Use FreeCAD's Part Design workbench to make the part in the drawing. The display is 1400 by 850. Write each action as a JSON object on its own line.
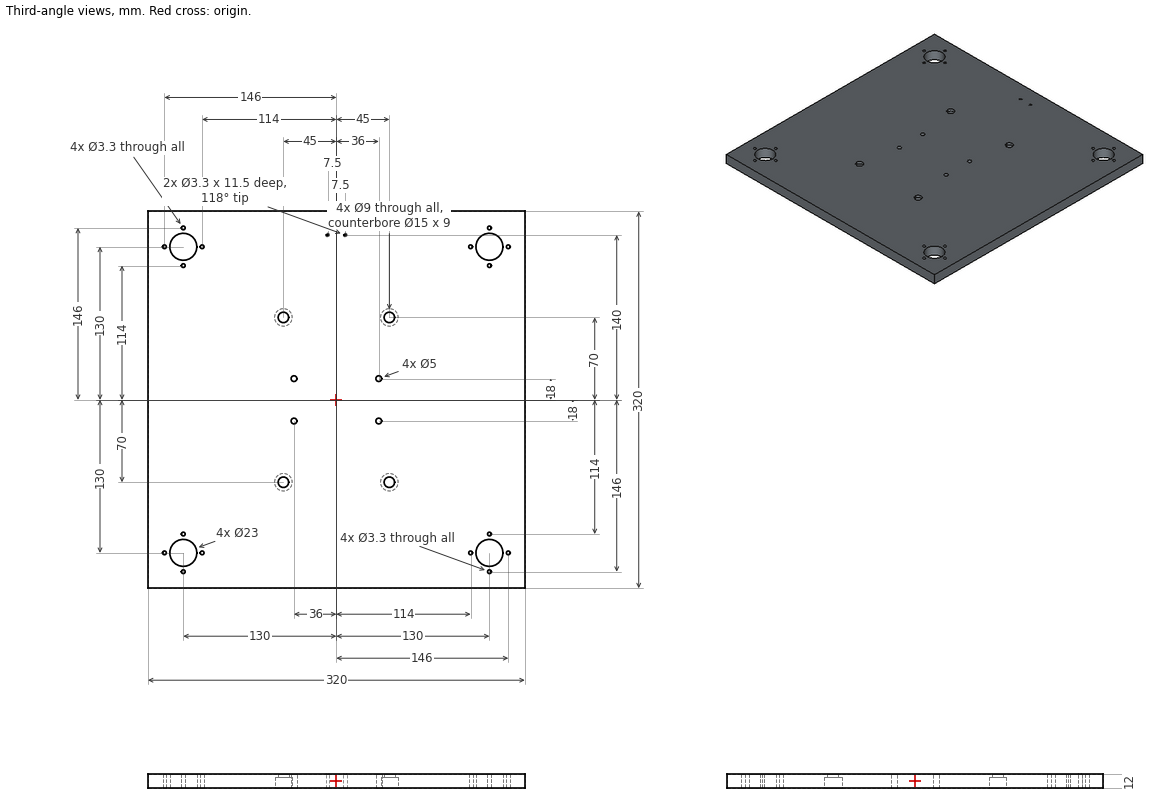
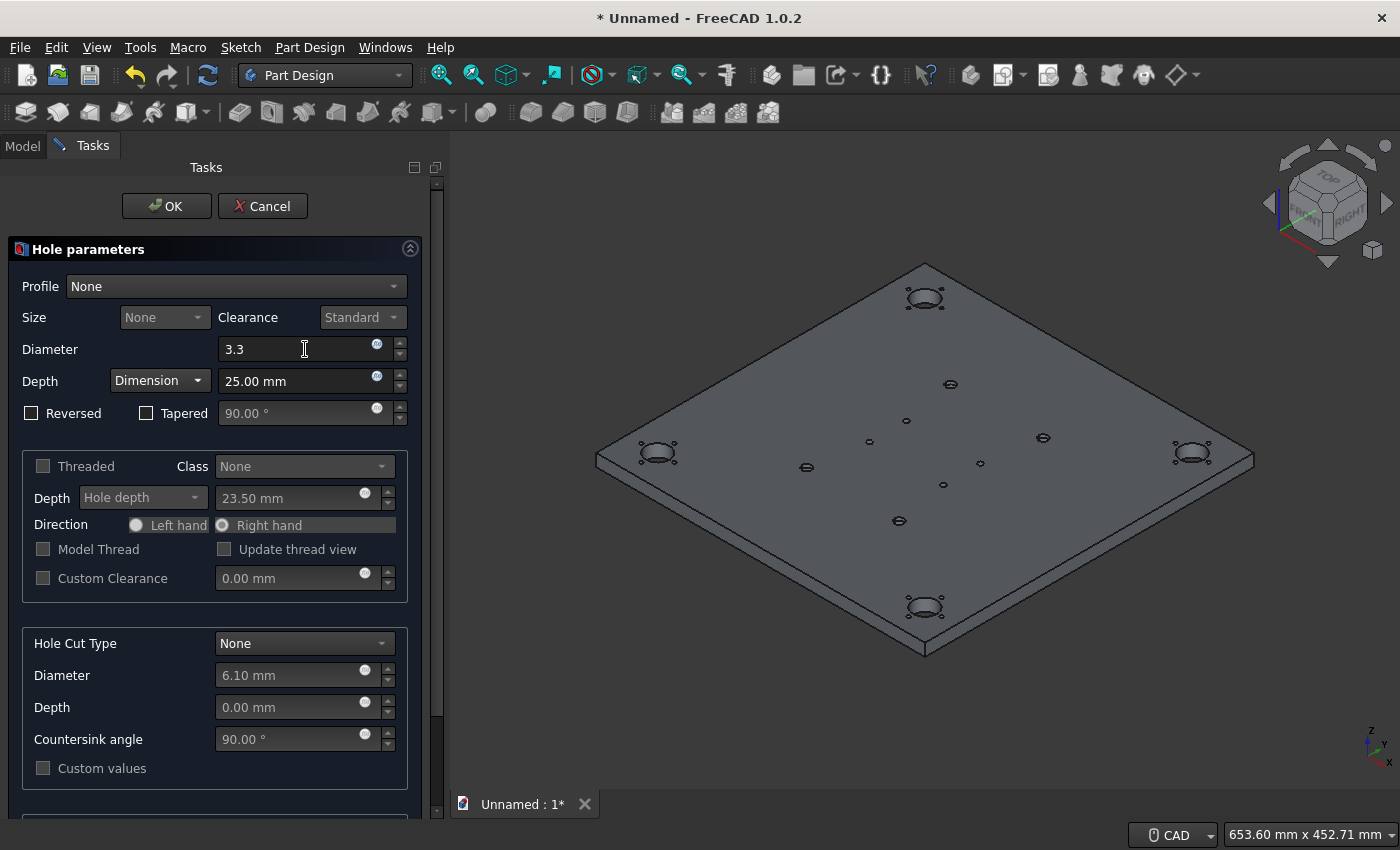
{"action": "left_click", "coordinate": [161, 380]}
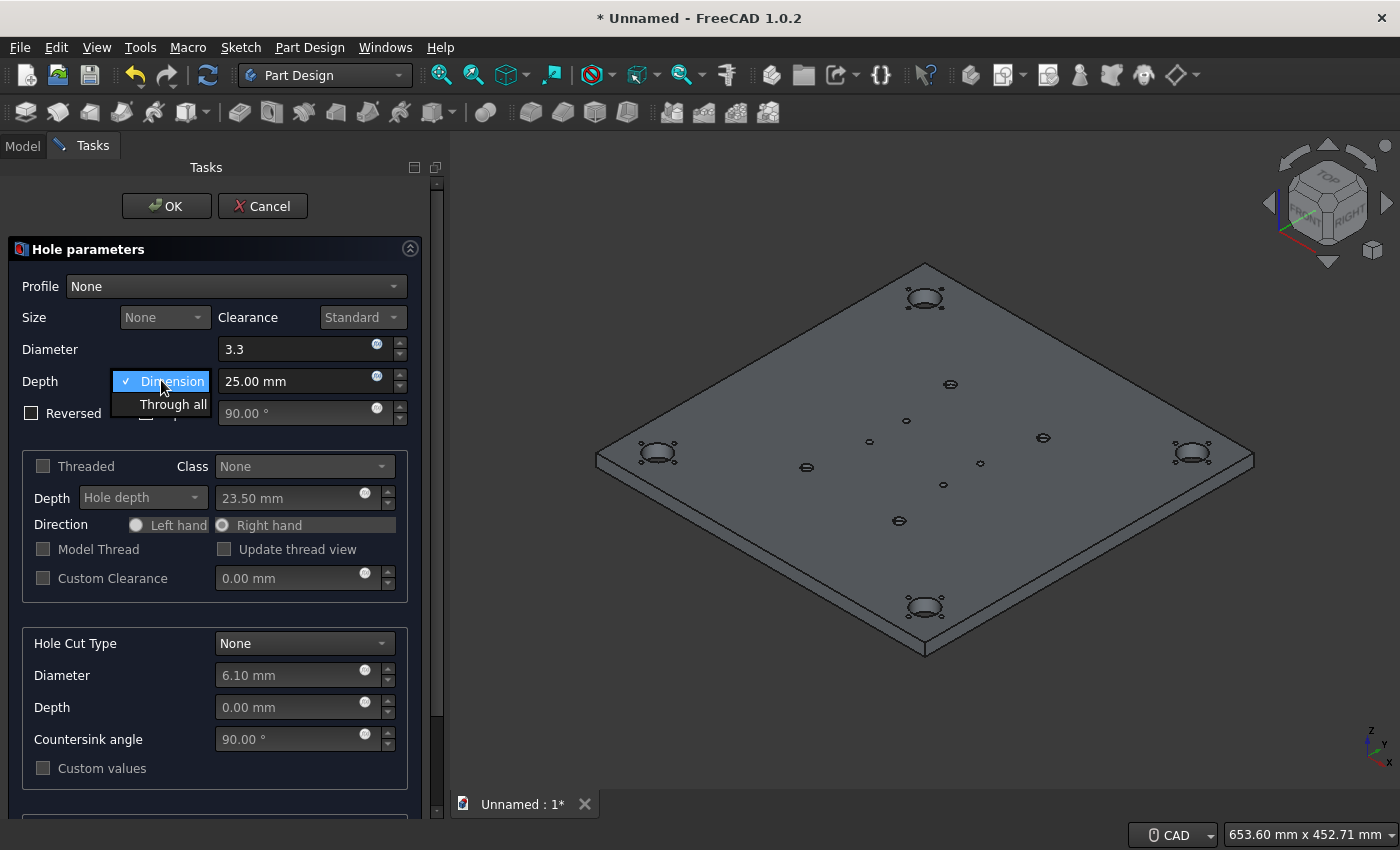
{"action": "left_click", "coordinate": [160, 404]}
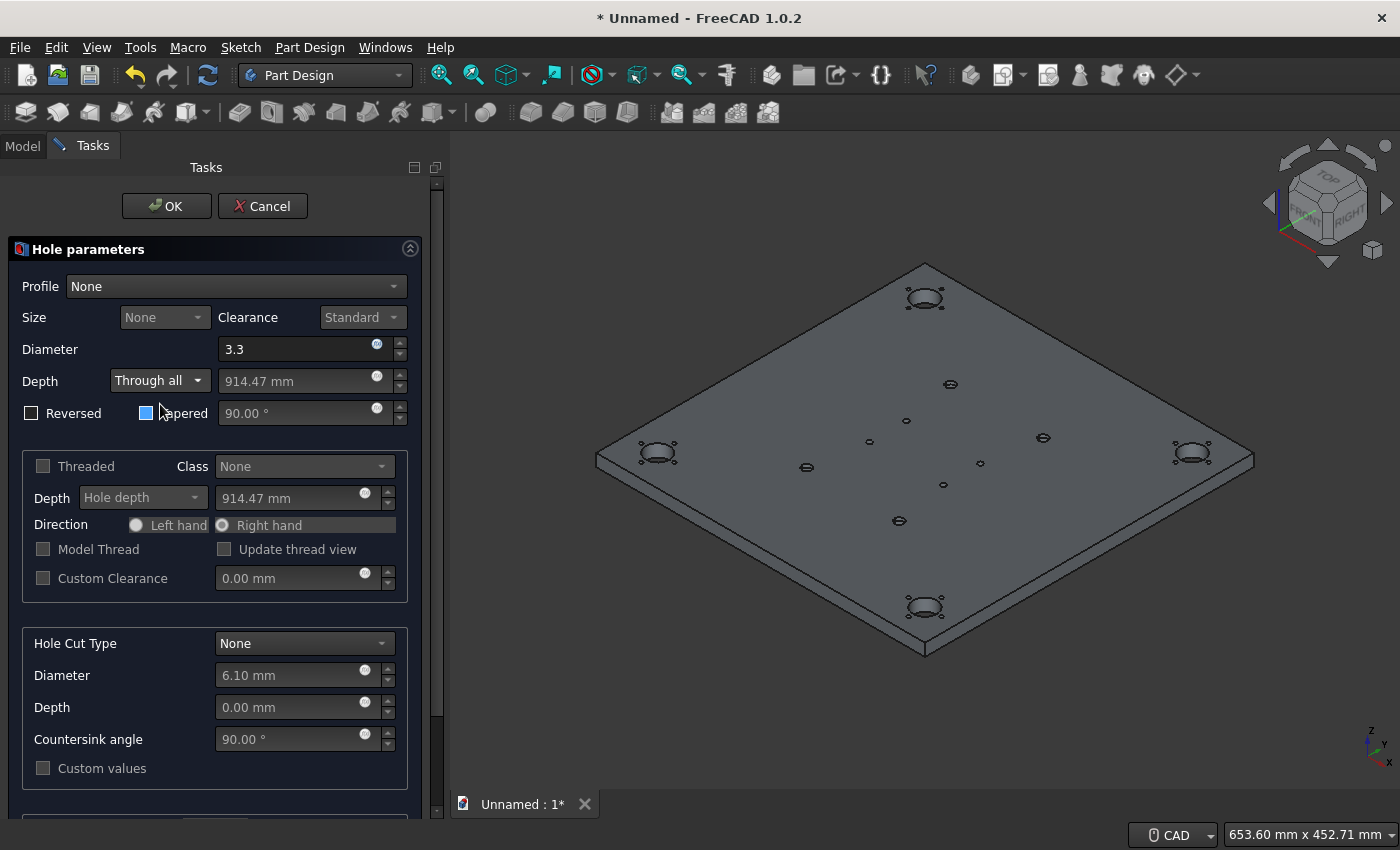
{"action": "left_click", "coordinate": [167, 206]}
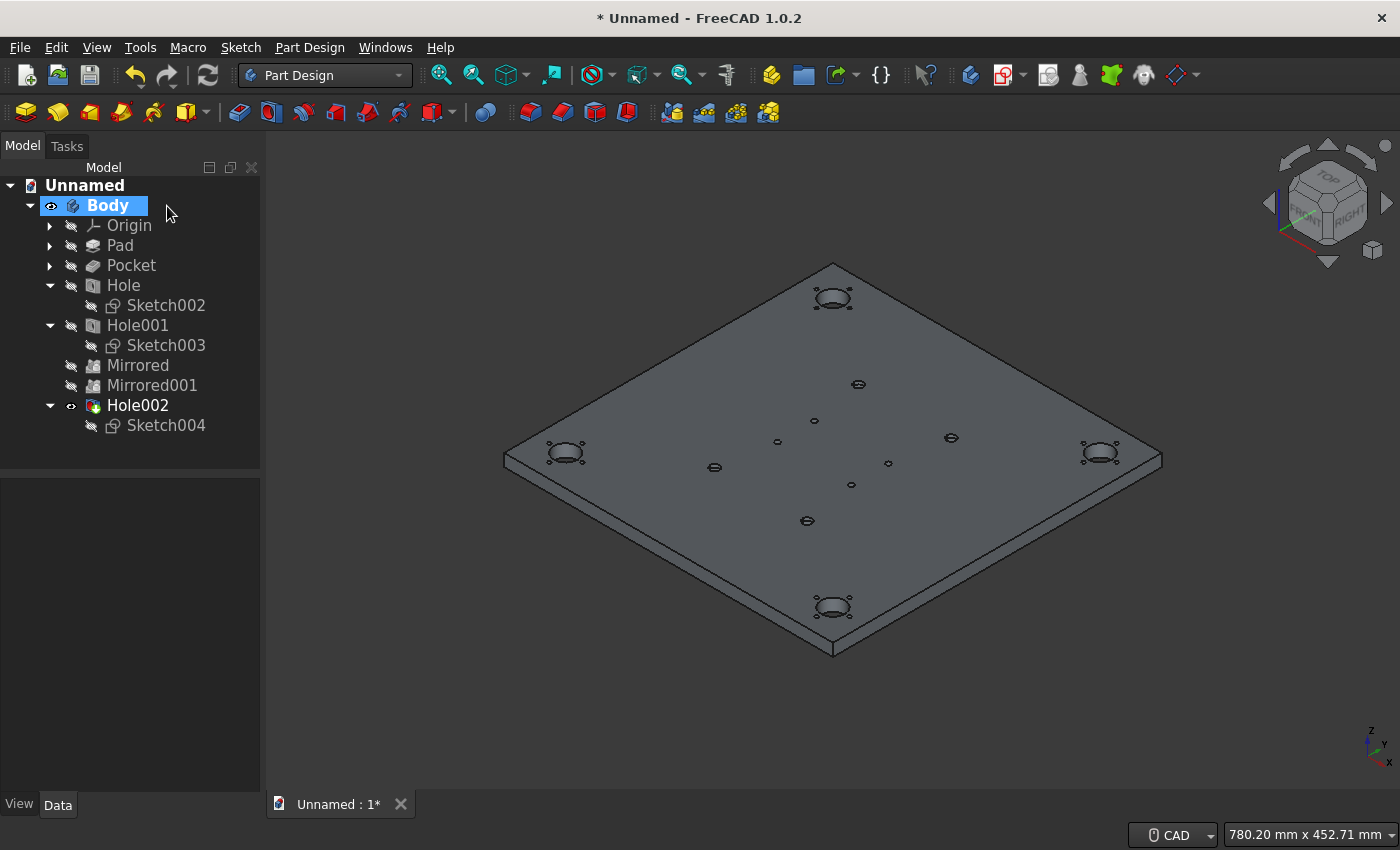
{"action": "key", "text": "5"}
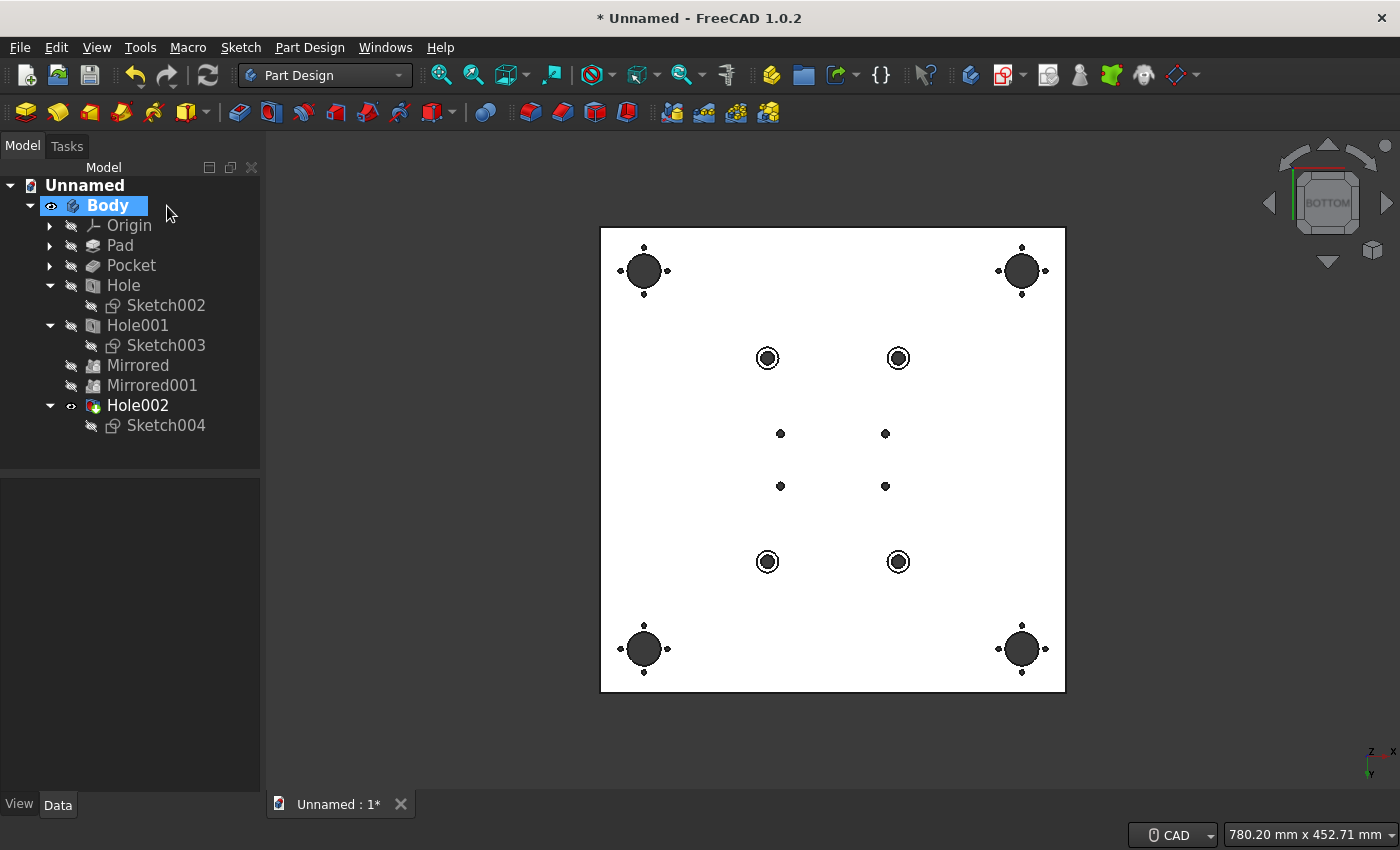
{"action": "left_click", "coordinate": [700, 459]}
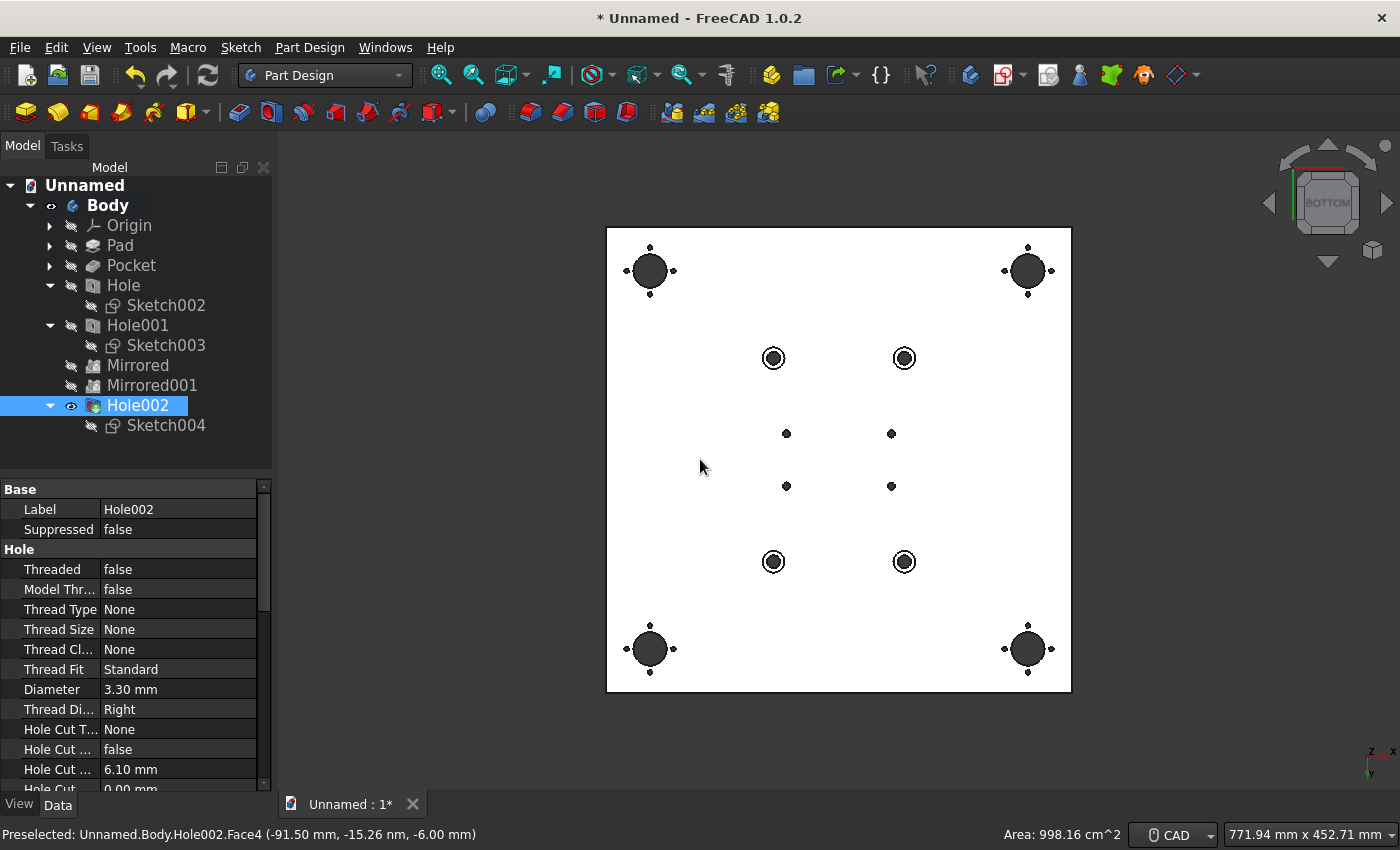
{"action": "left_click", "coordinate": [1004, 76]}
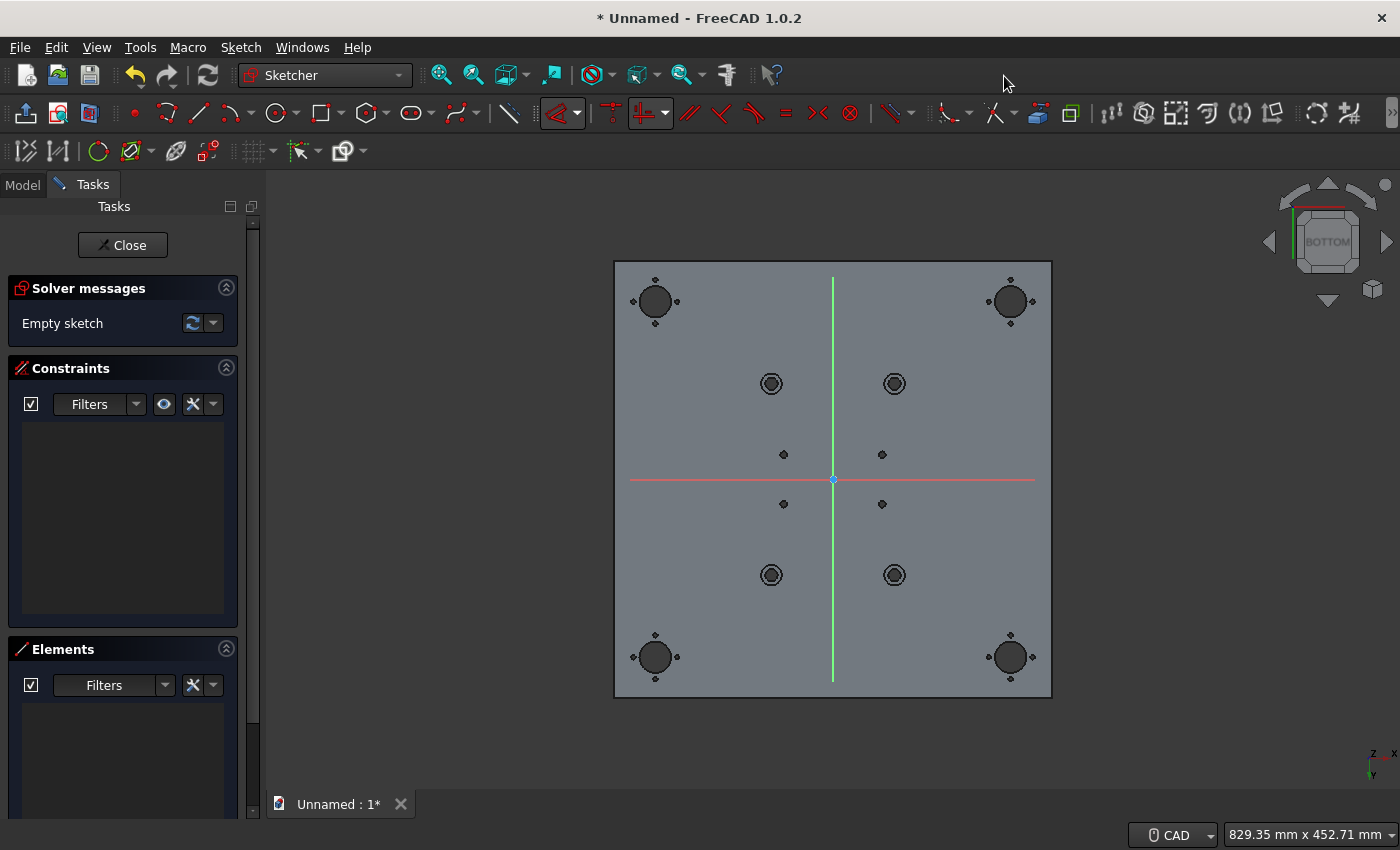
{"action": "scroll", "coordinate": [837, 681], "scroll_direction": "up", "scroll_amount": 15}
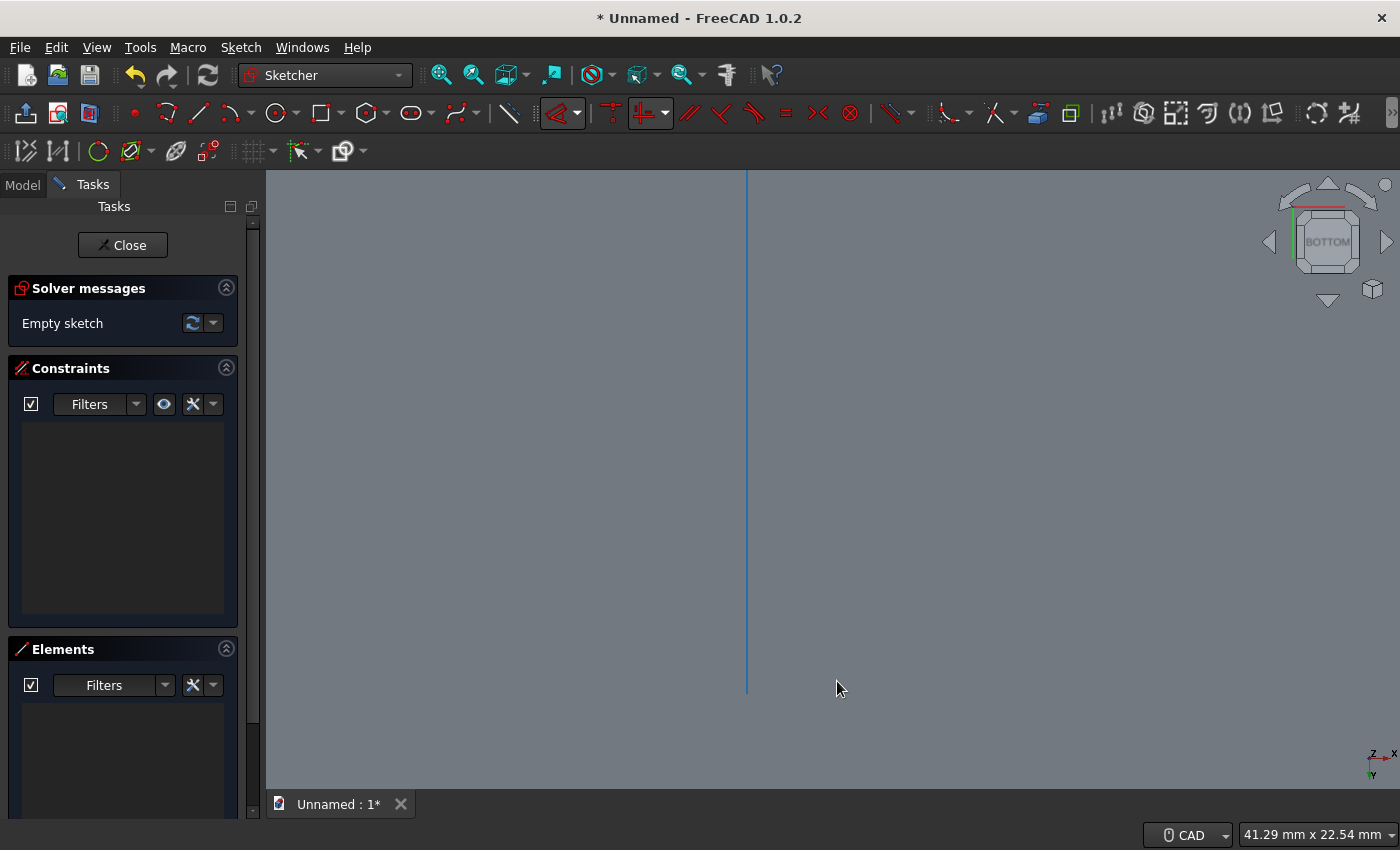
{"action": "left_click", "coordinate": [276, 114]}